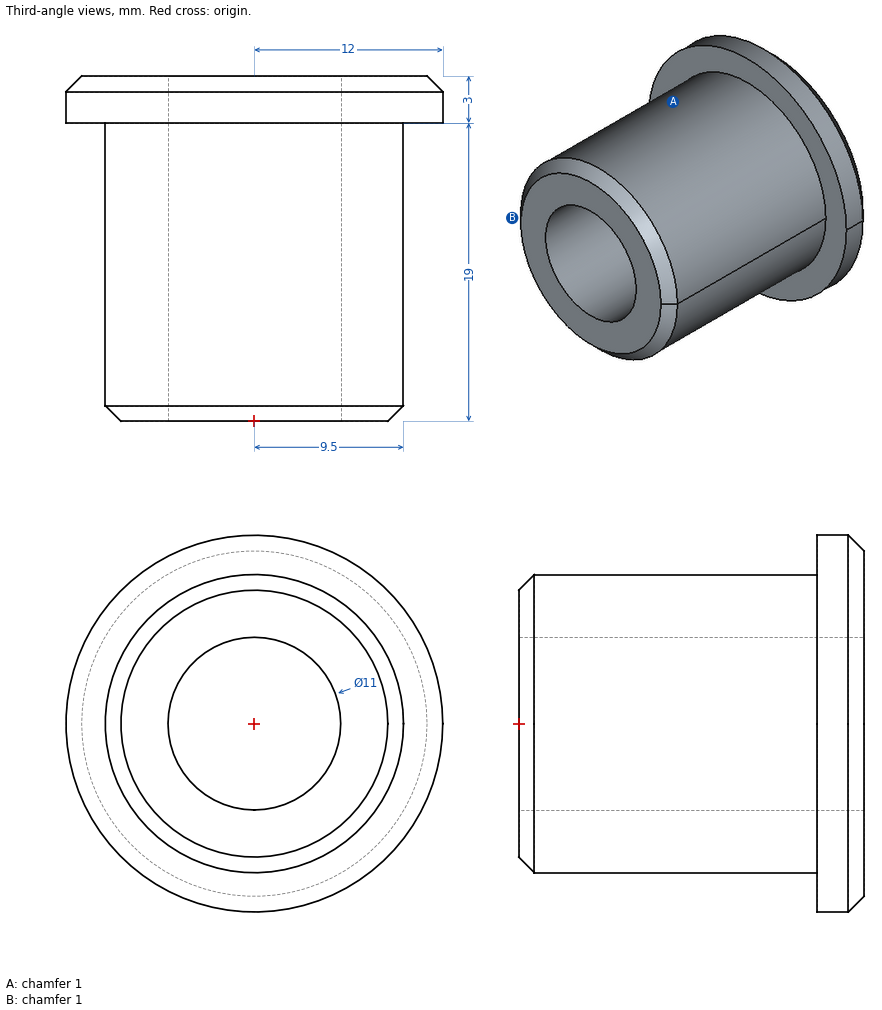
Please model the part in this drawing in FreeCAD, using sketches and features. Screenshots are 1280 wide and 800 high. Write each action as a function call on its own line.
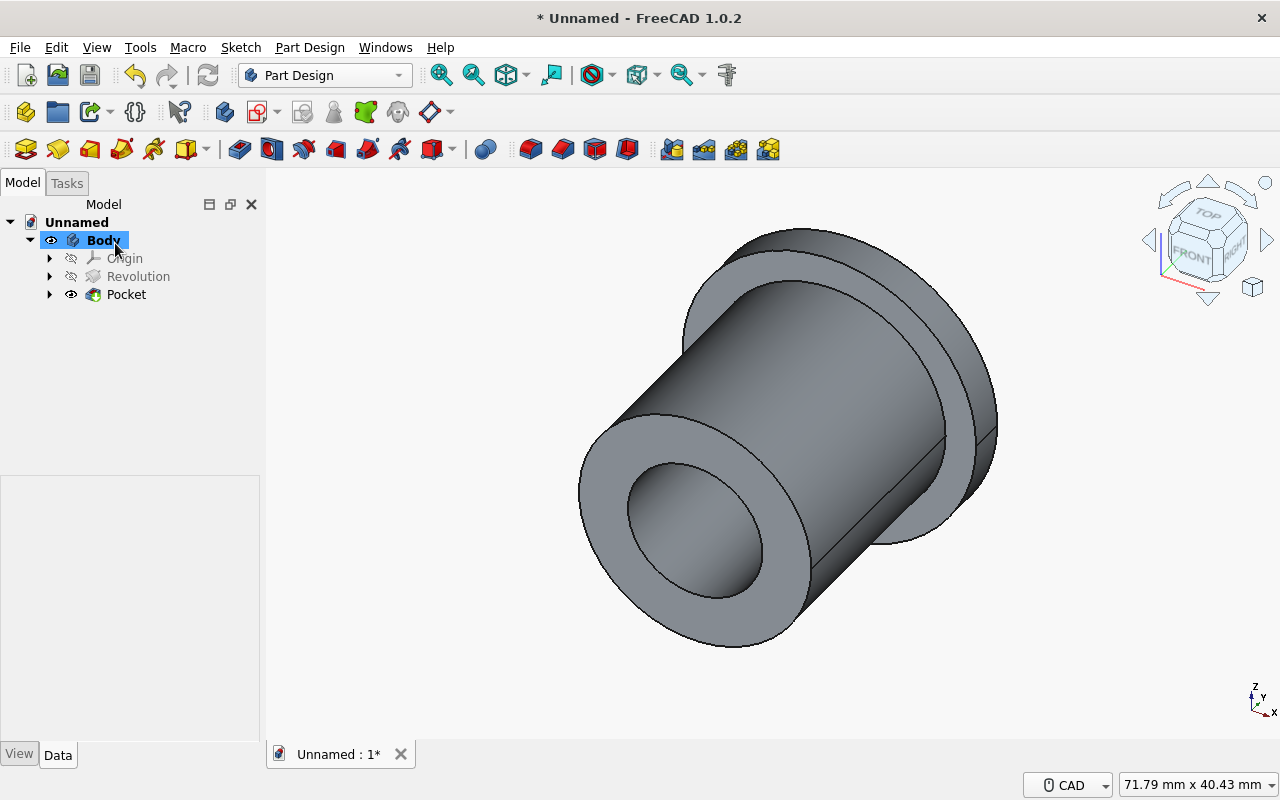
click(896, 258)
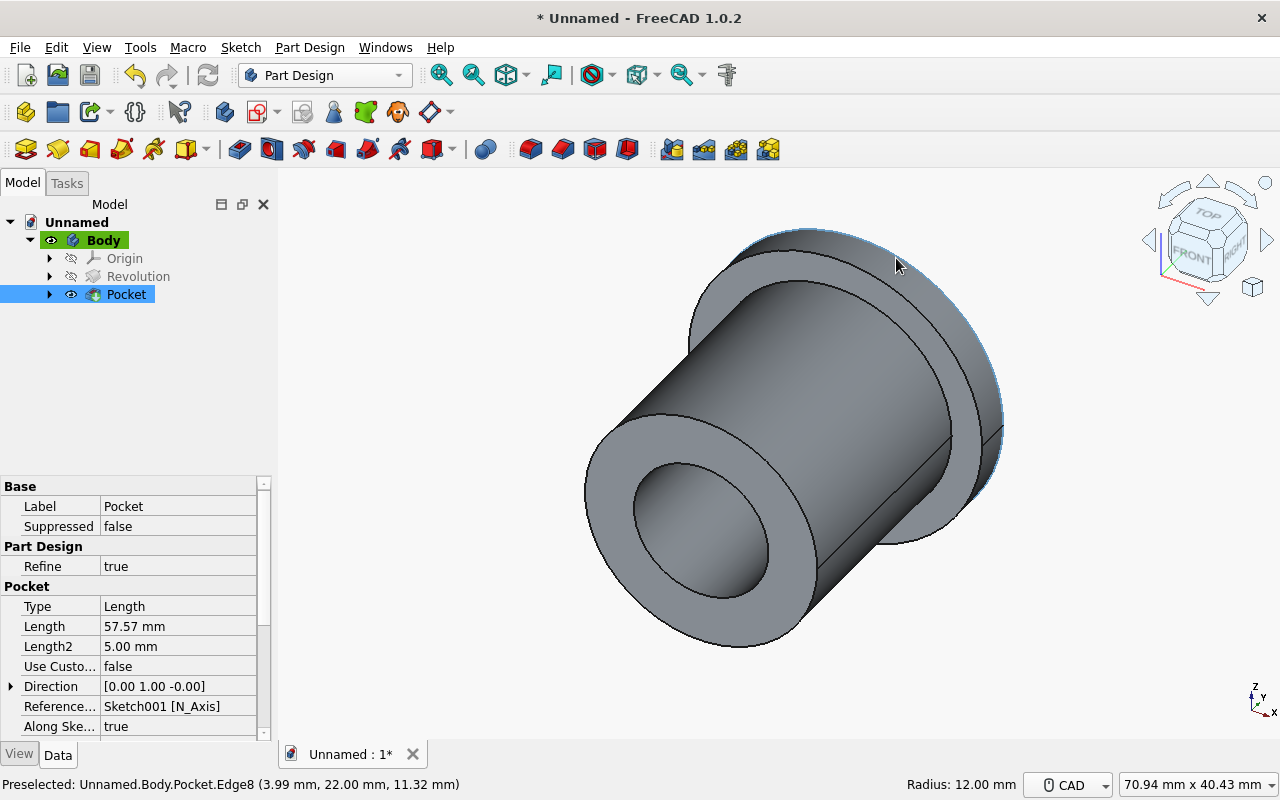
click(564, 150)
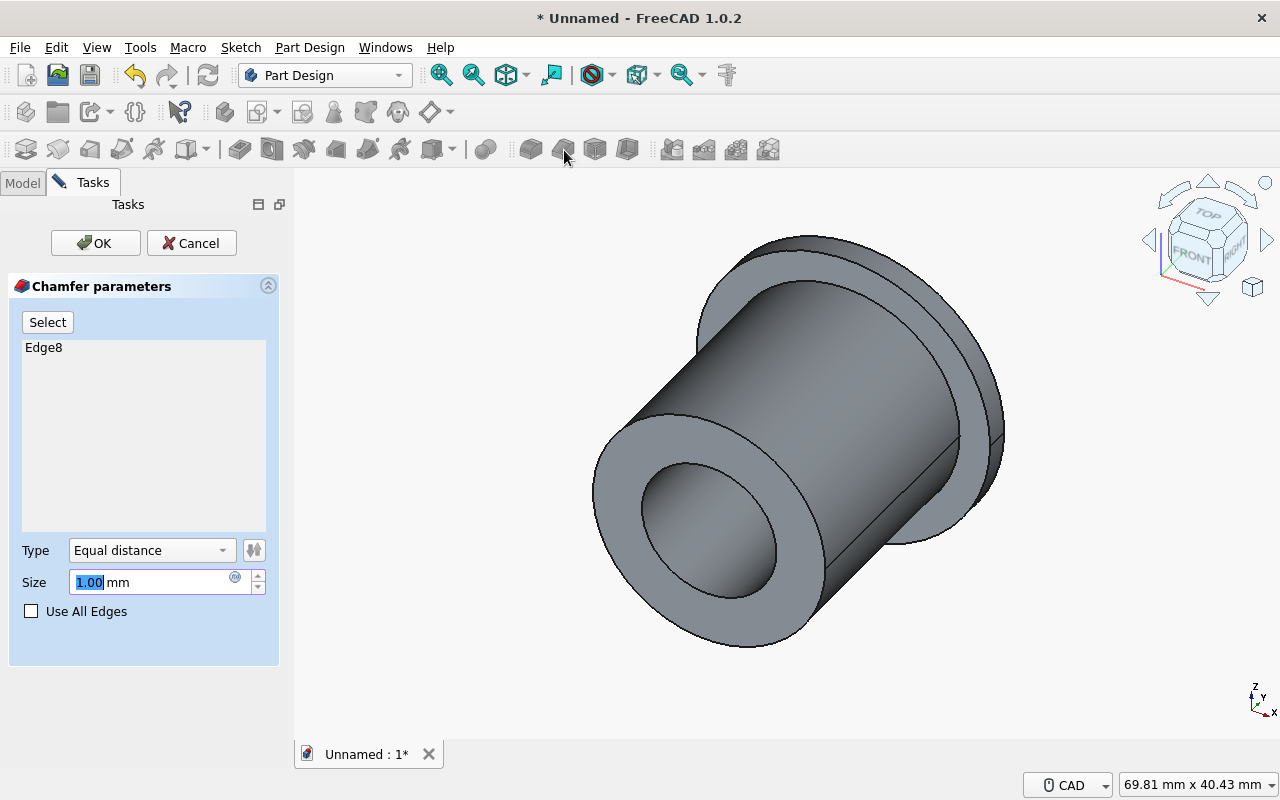
text(1)
key(Tab)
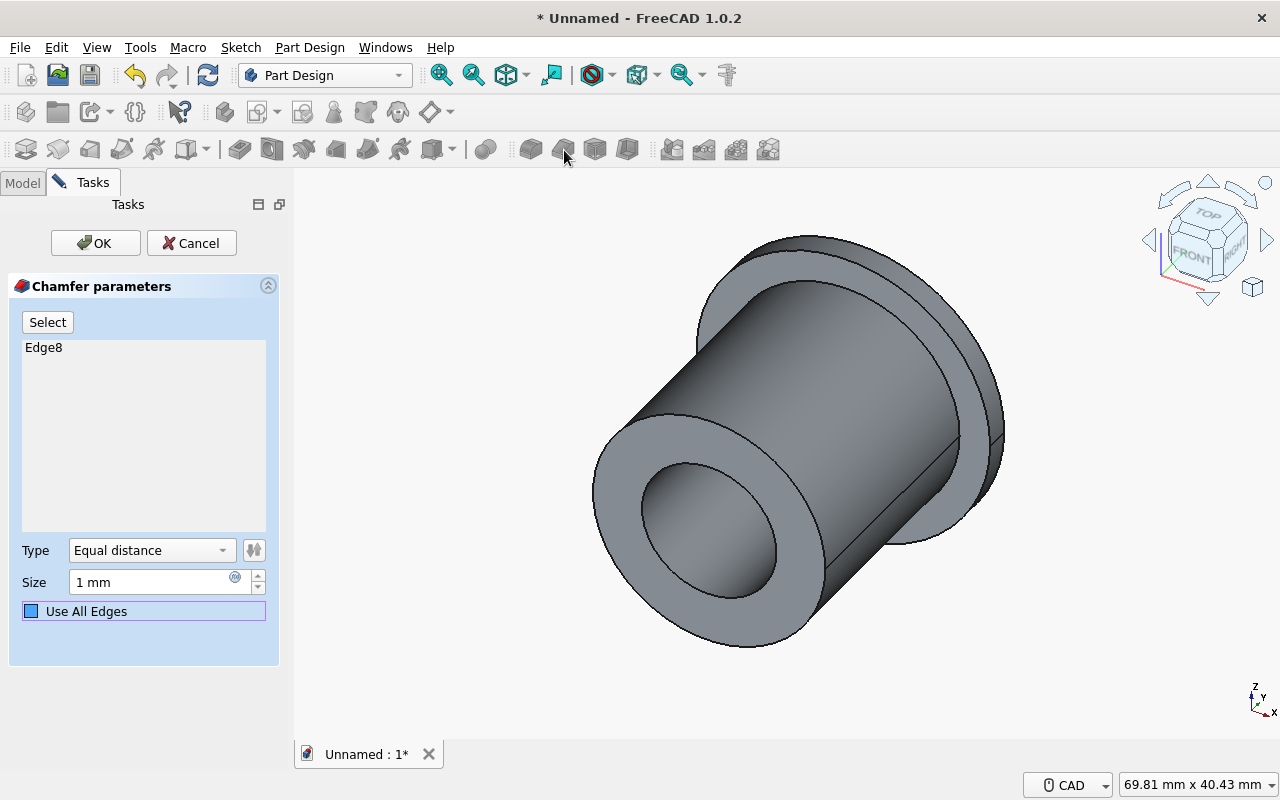
click(96, 243)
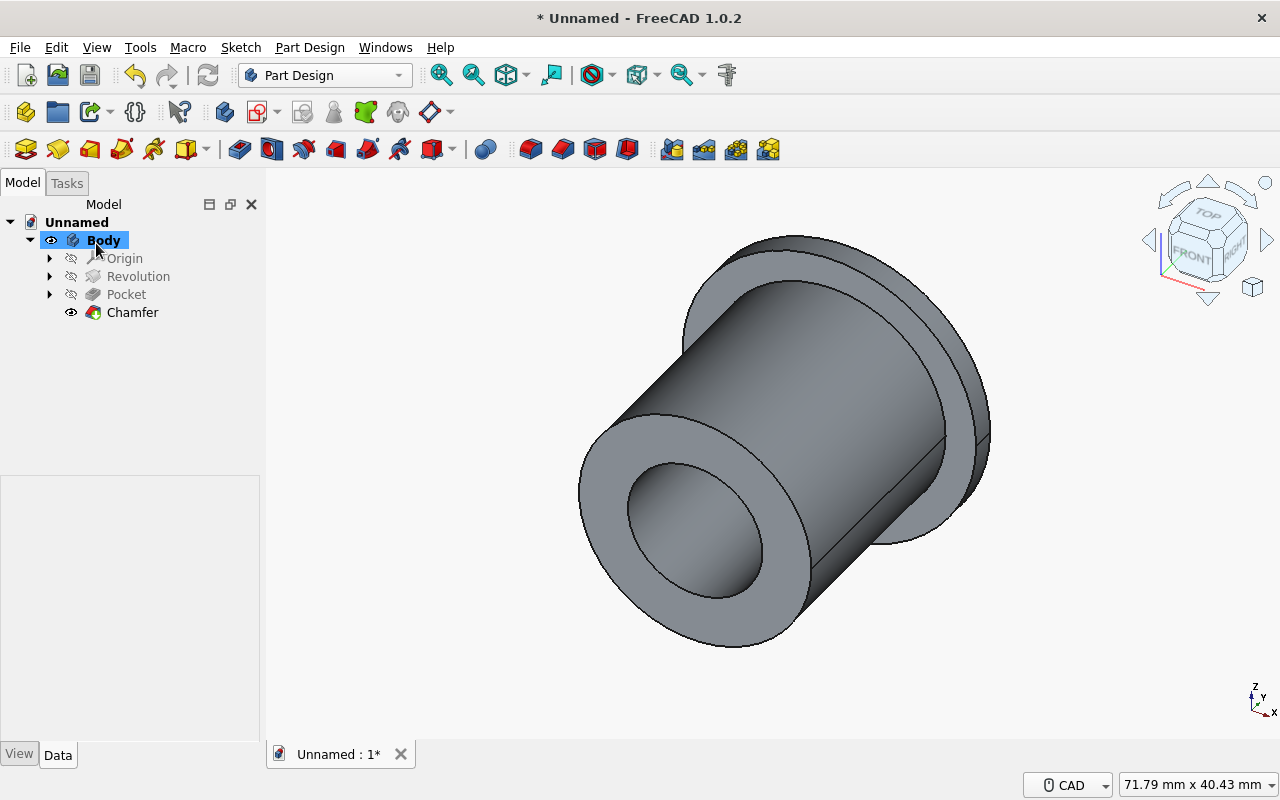
click(601, 434)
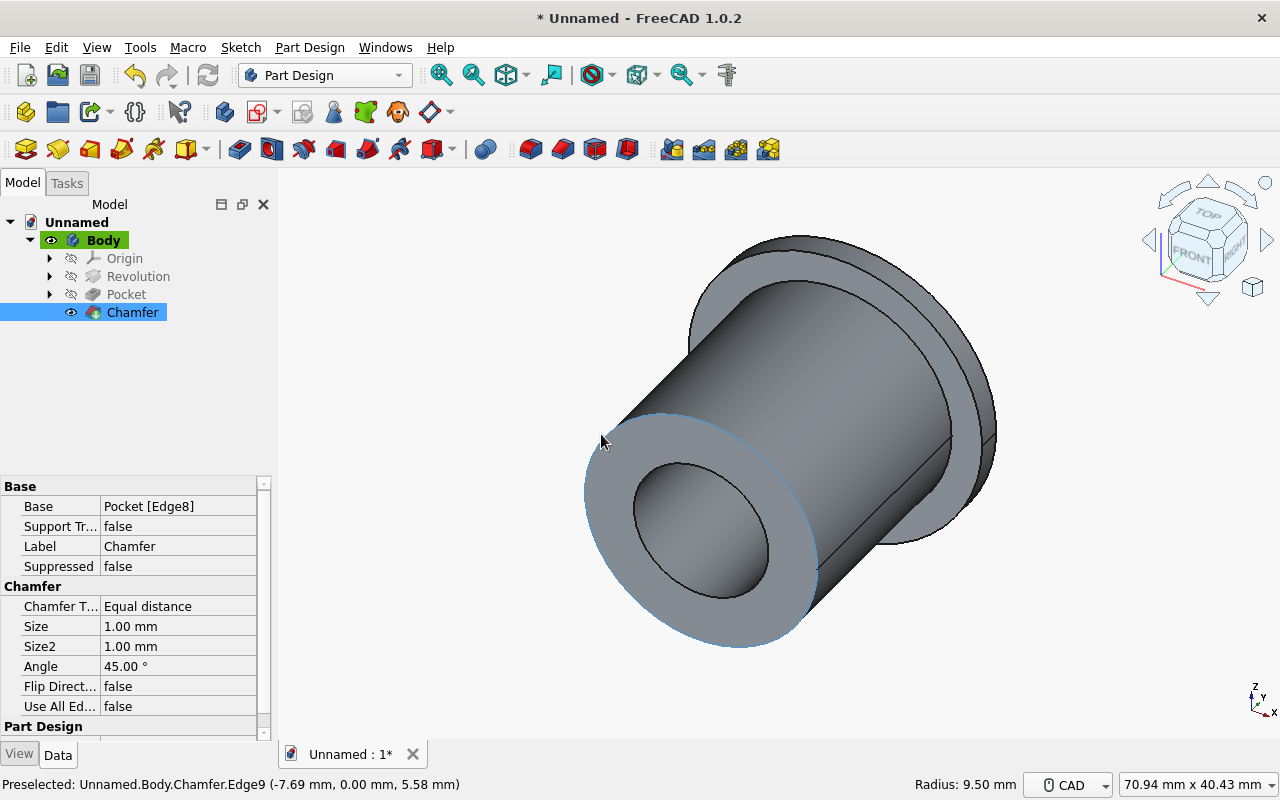
click(564, 150)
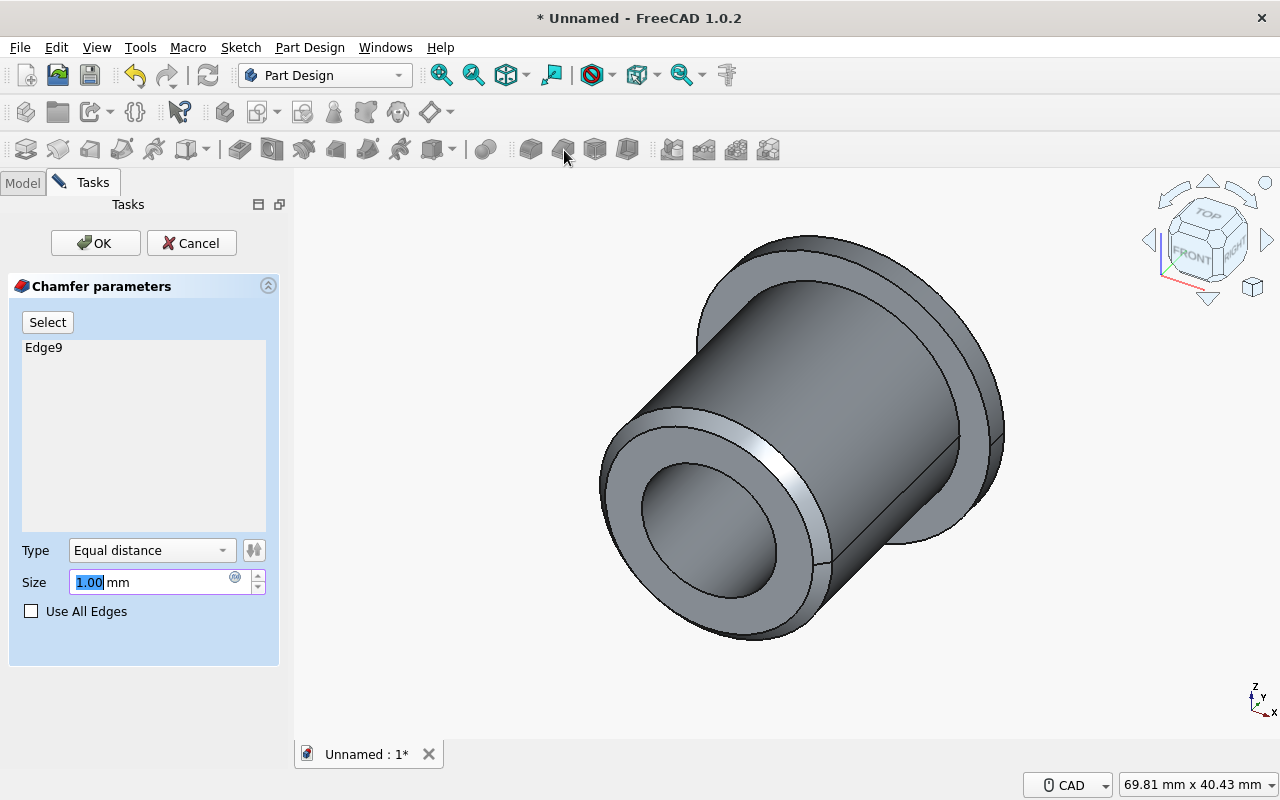
text(1)
key(Tab)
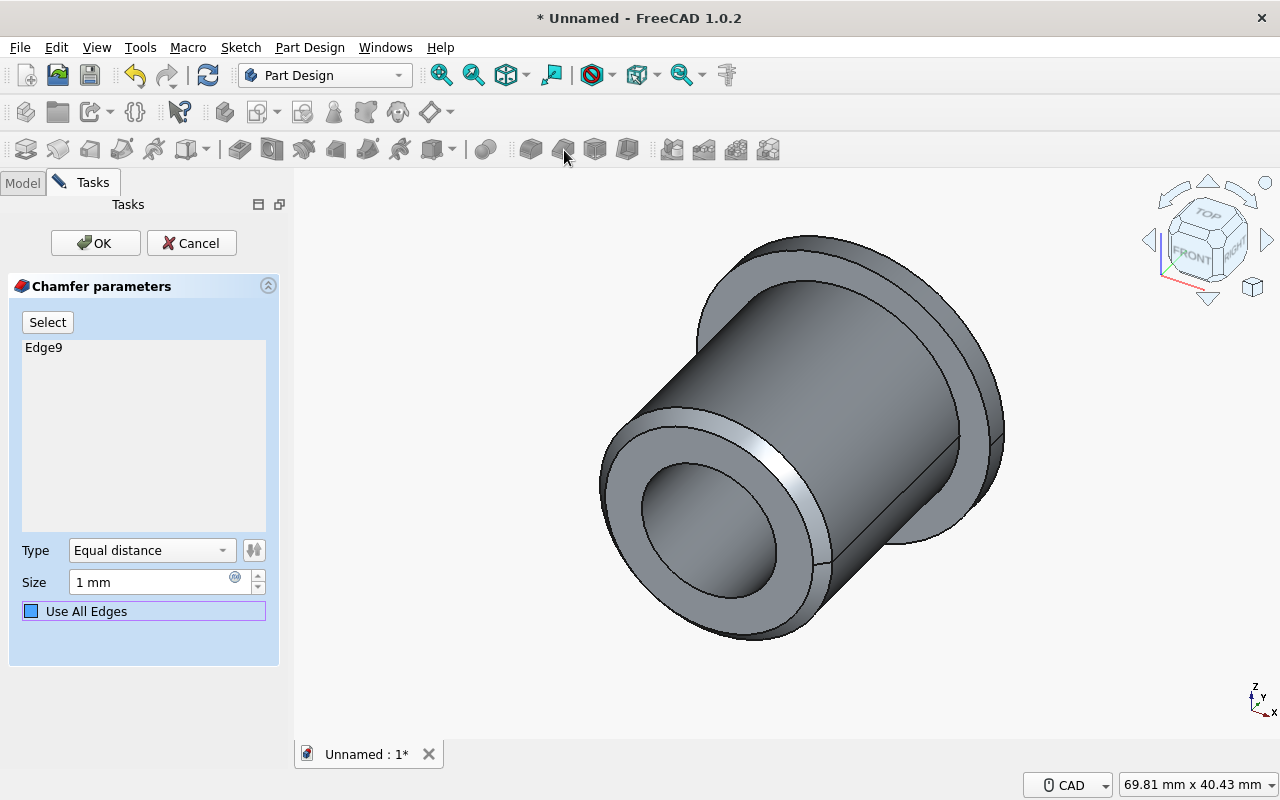
click(96, 243)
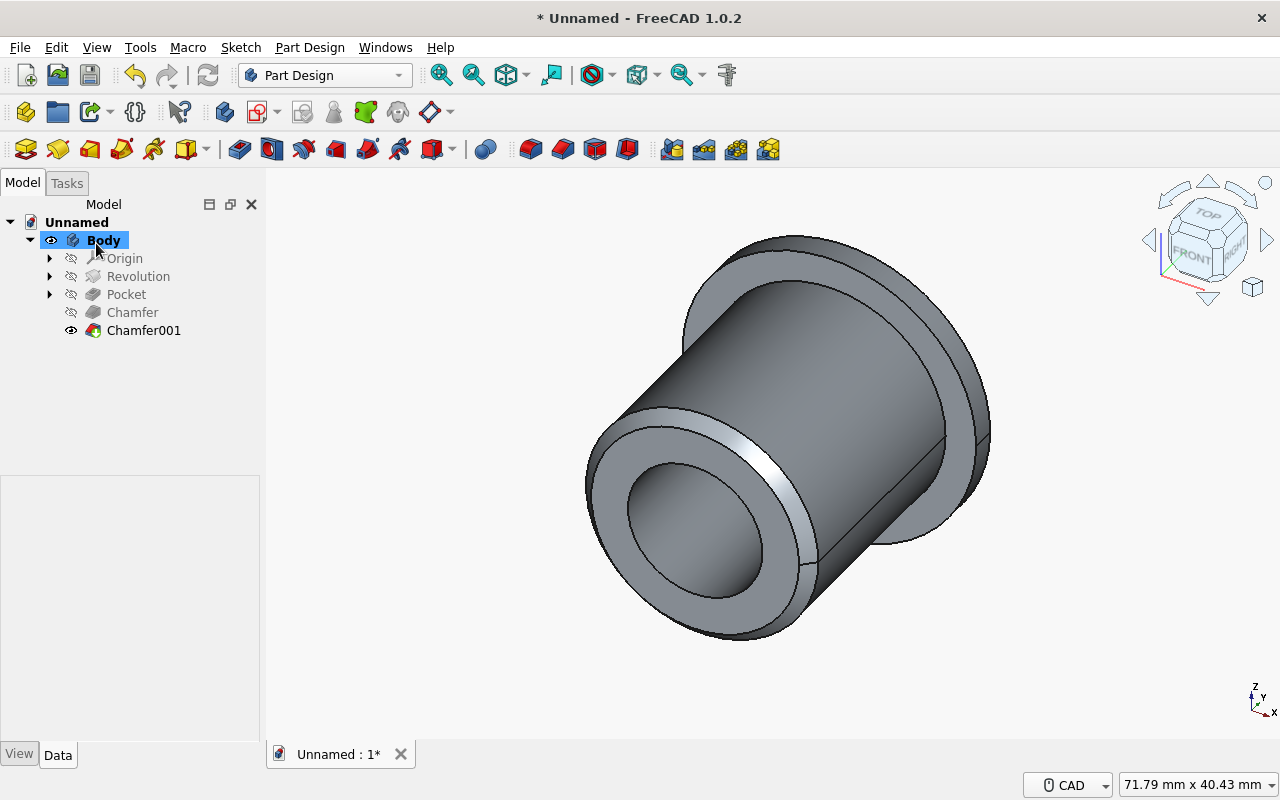
key(0)